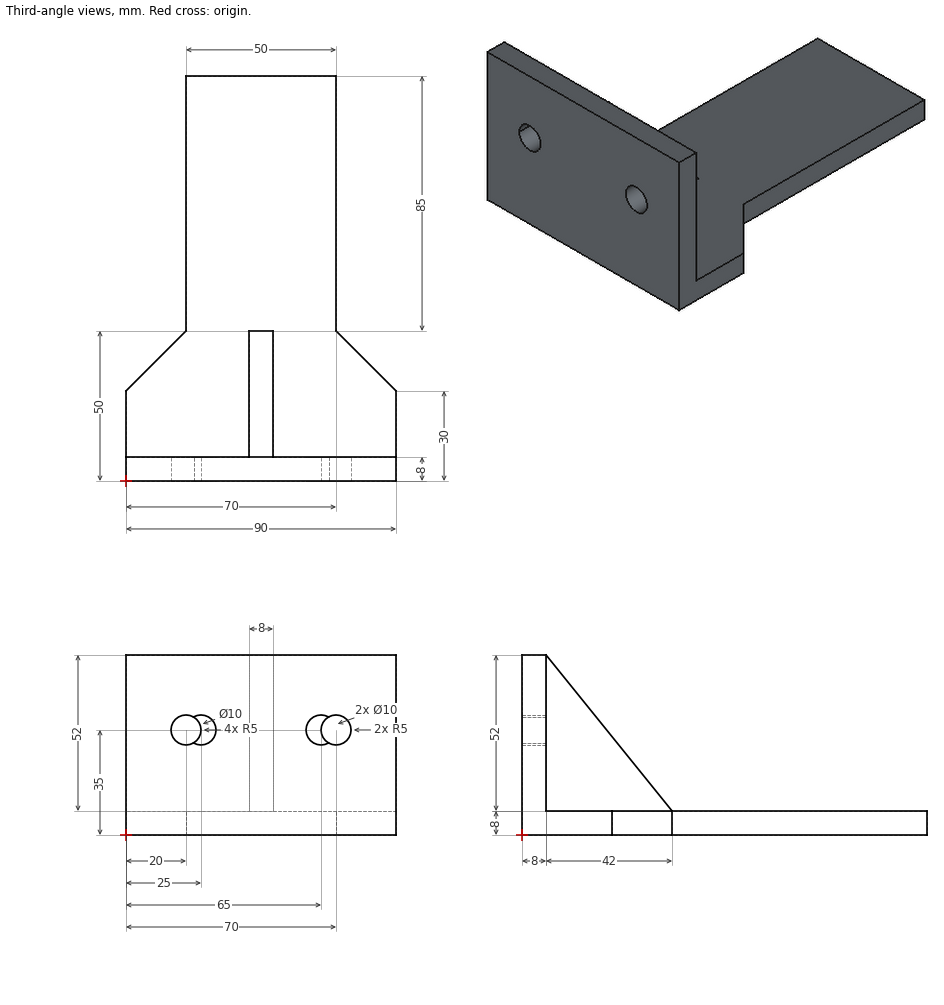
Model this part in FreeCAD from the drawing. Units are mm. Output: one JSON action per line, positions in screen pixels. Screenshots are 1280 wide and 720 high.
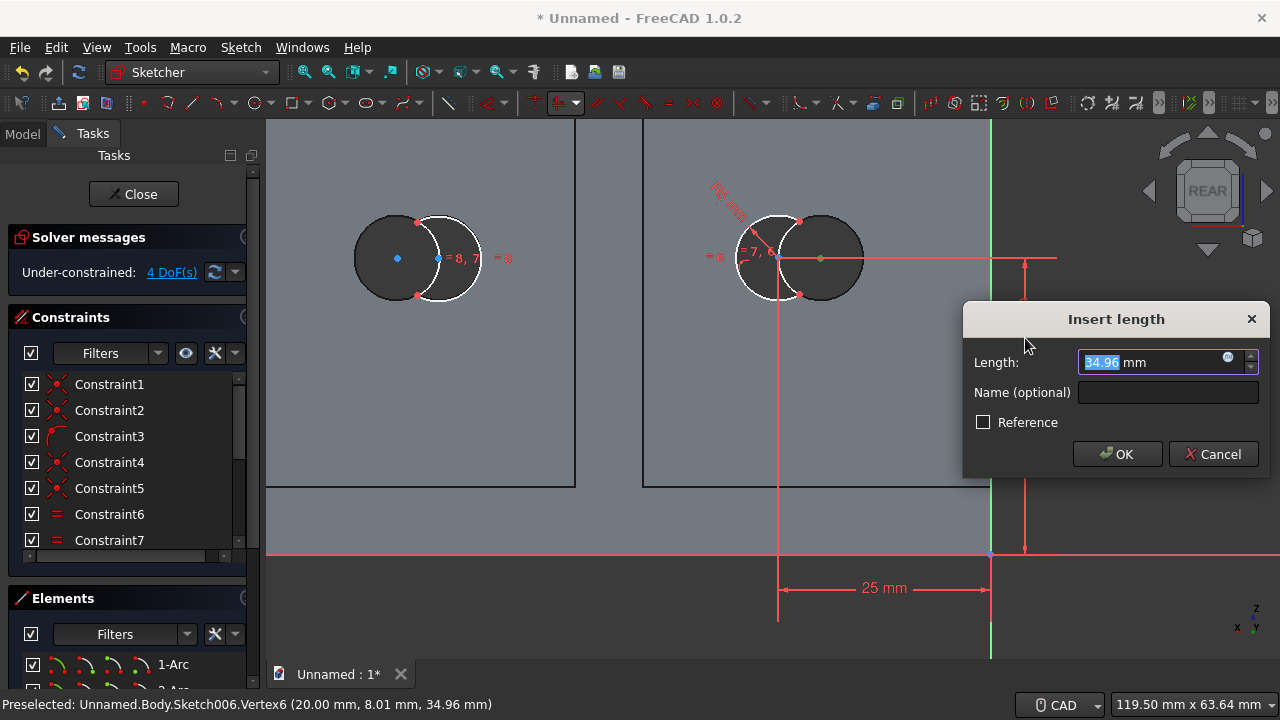
{"action": "type", "text": "35"}
{"action": "key", "text": "Return"}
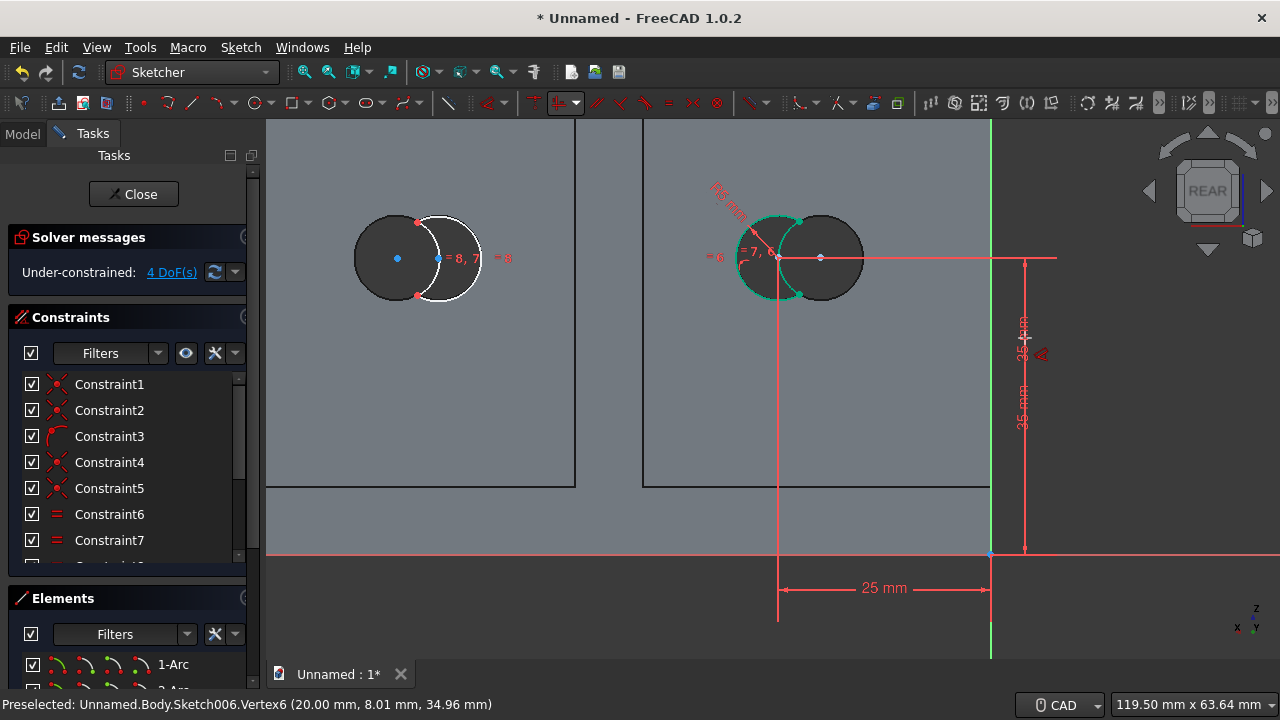
{"action": "left_click", "coordinate": [397, 259]}
{"action": "left_click", "coordinate": [694, 589]}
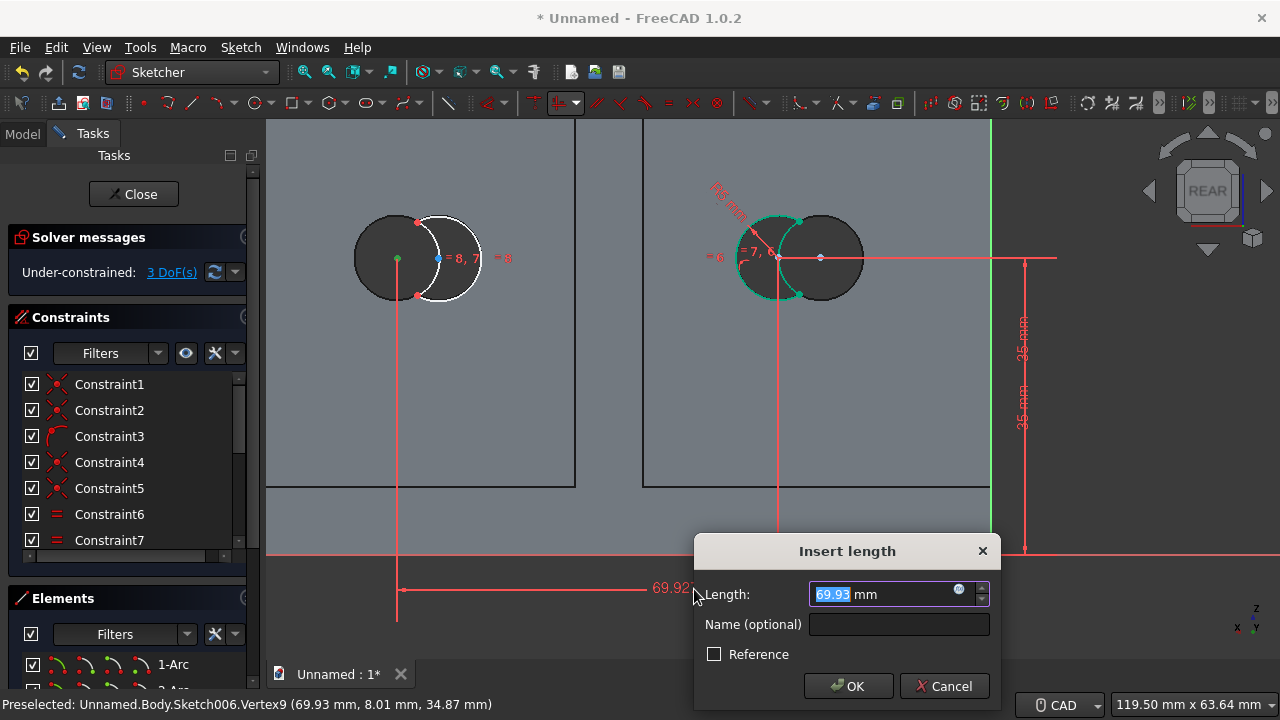
{"action": "type", "text": "70"}
{"action": "key", "text": "Return"}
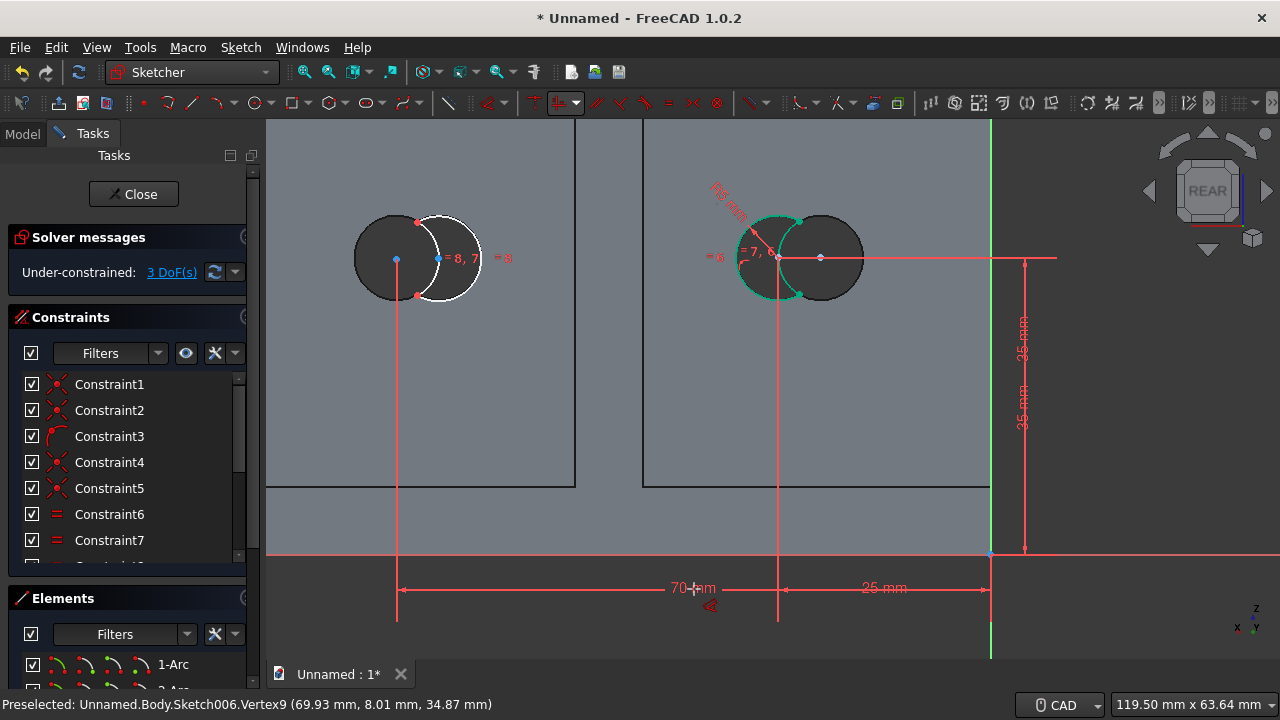
{"action": "left_click", "coordinate": [397, 259]}
{"action": "left_click", "coordinate": [363, 407]}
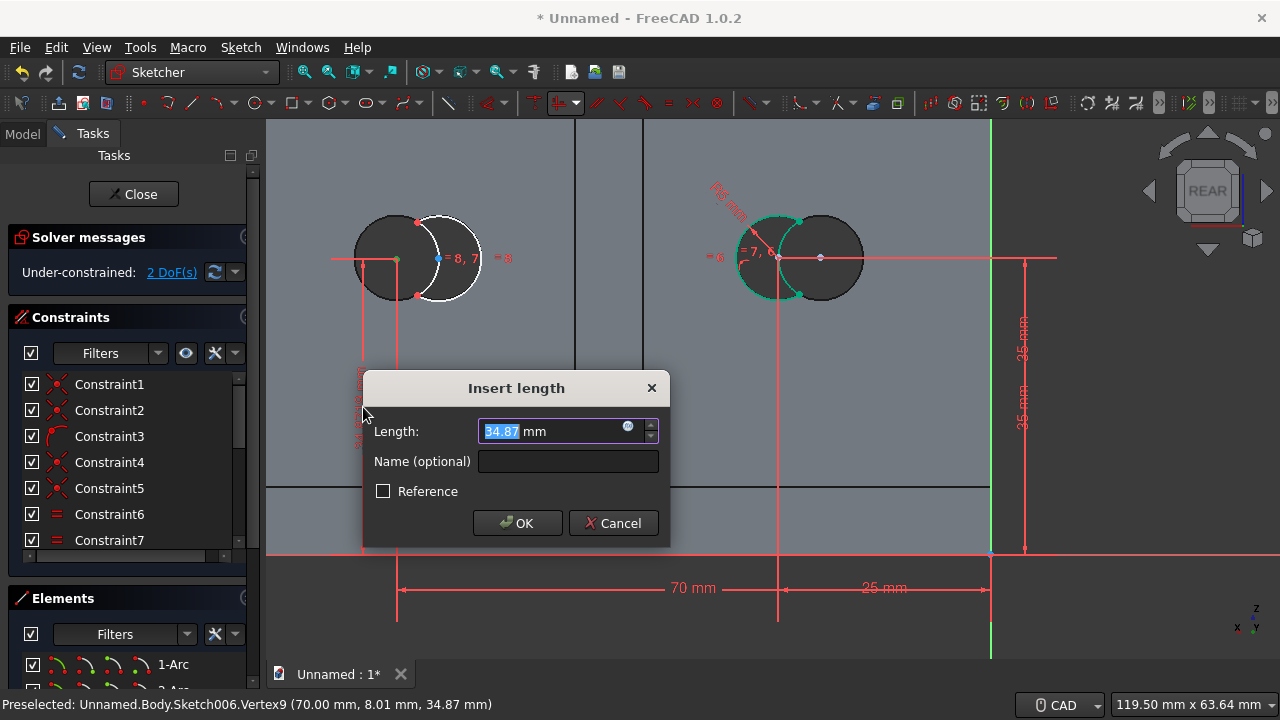
{"action": "type", "text": "35"}
{"action": "key", "text": "Return"}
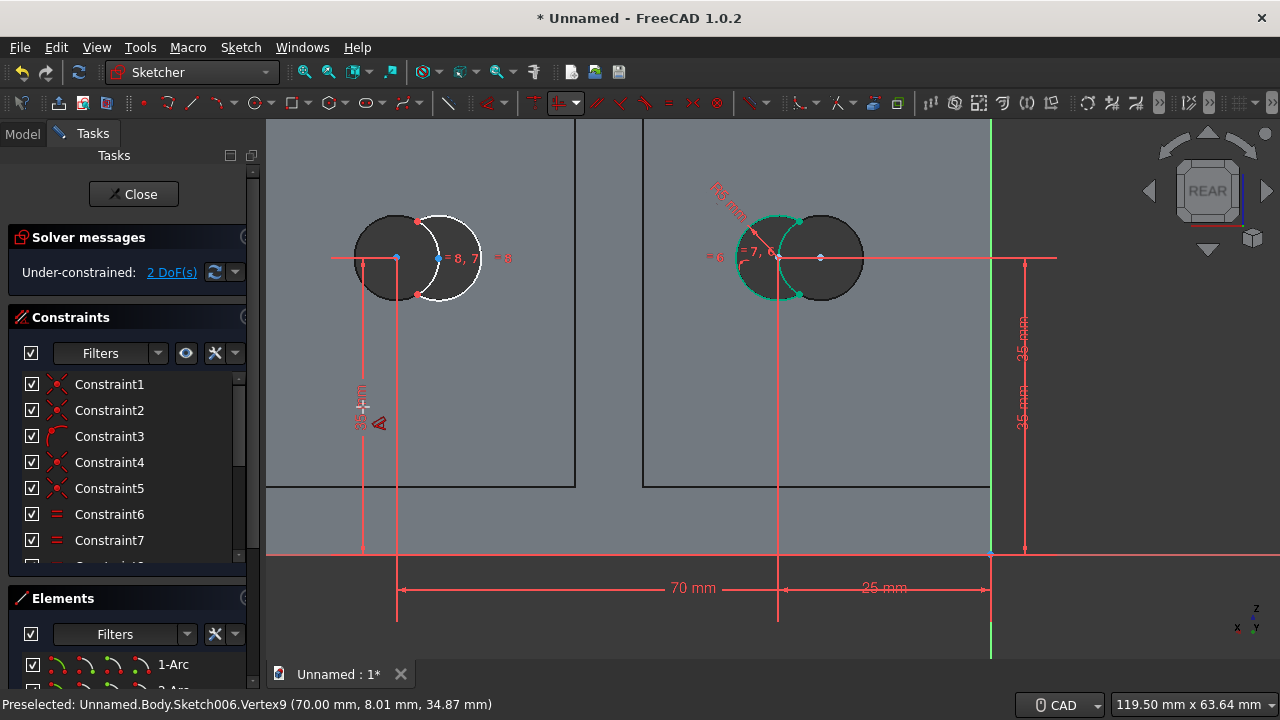
{"action": "left_click", "coordinate": [439, 258]}
{"action": "left_click", "coordinate": [588, 589]}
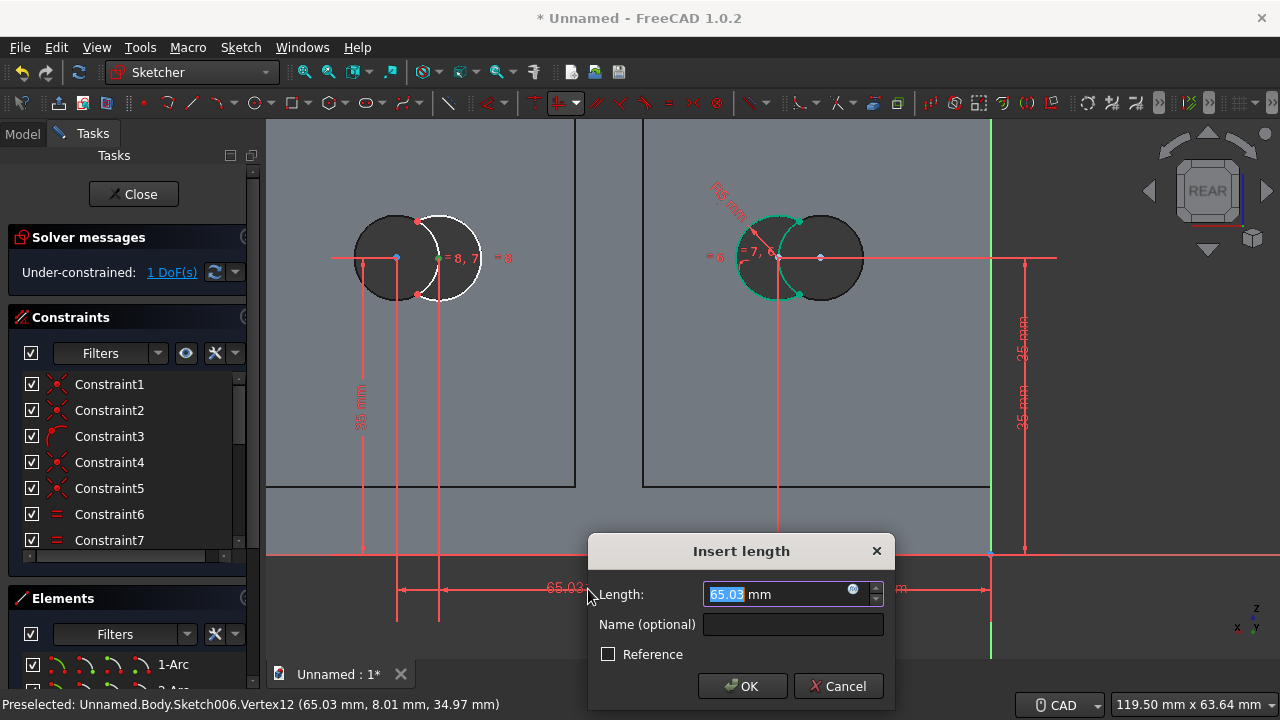
{"action": "type", "text": "65"}
{"action": "key", "text": "Return"}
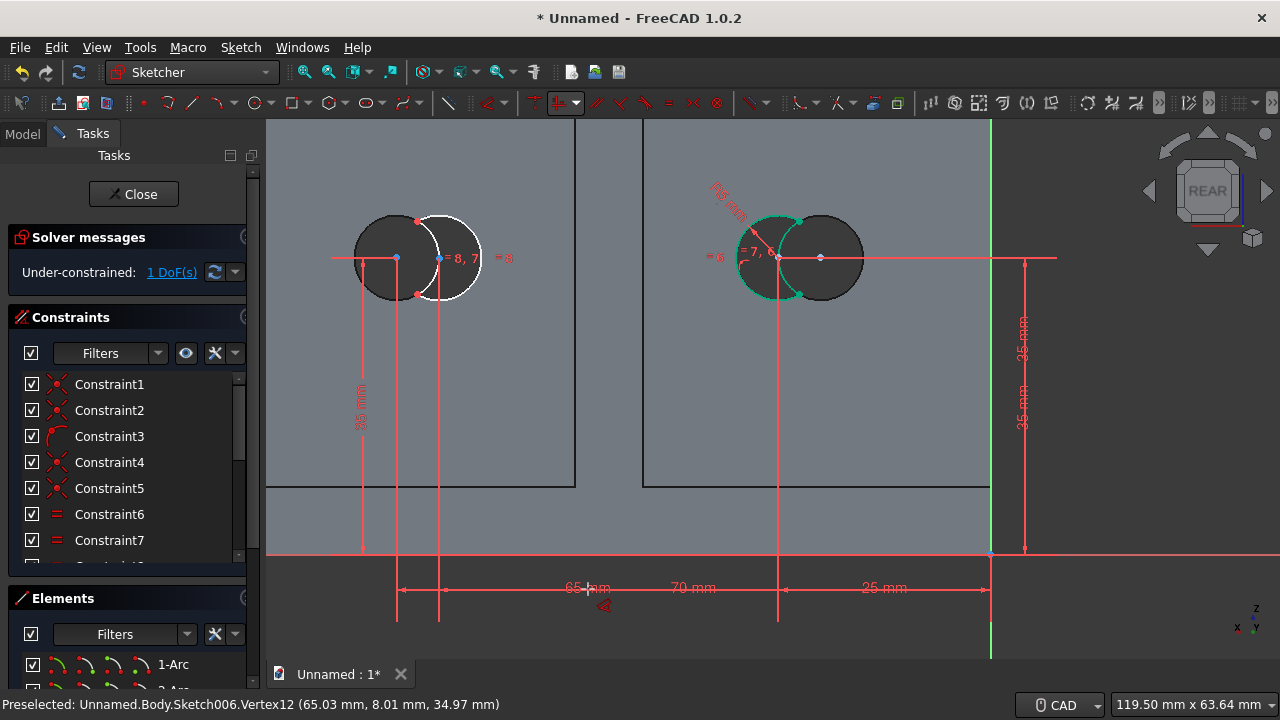
{"action": "left_click", "coordinate": [439, 258]}
{"action": "left_click", "coordinate": [1025, 475]}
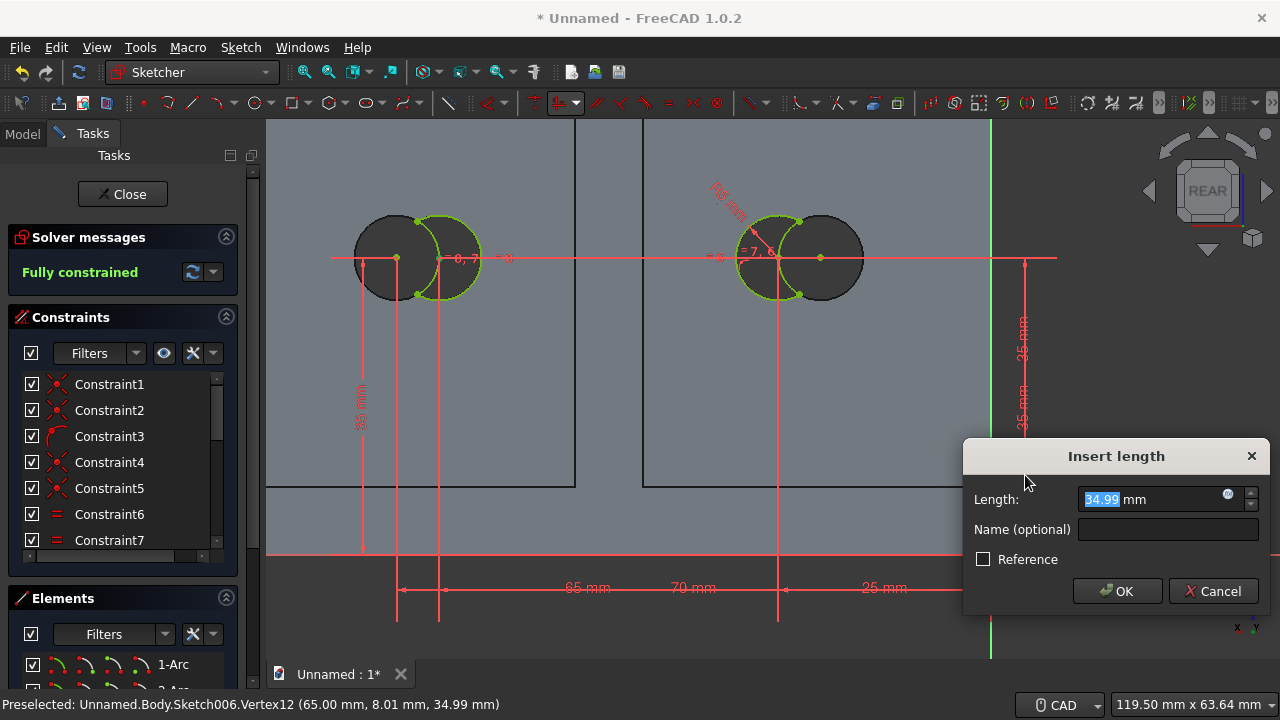
{"action": "type", "text": "35"}
{"action": "key", "text": "Return"}
{"action": "key", "text": "Escape"}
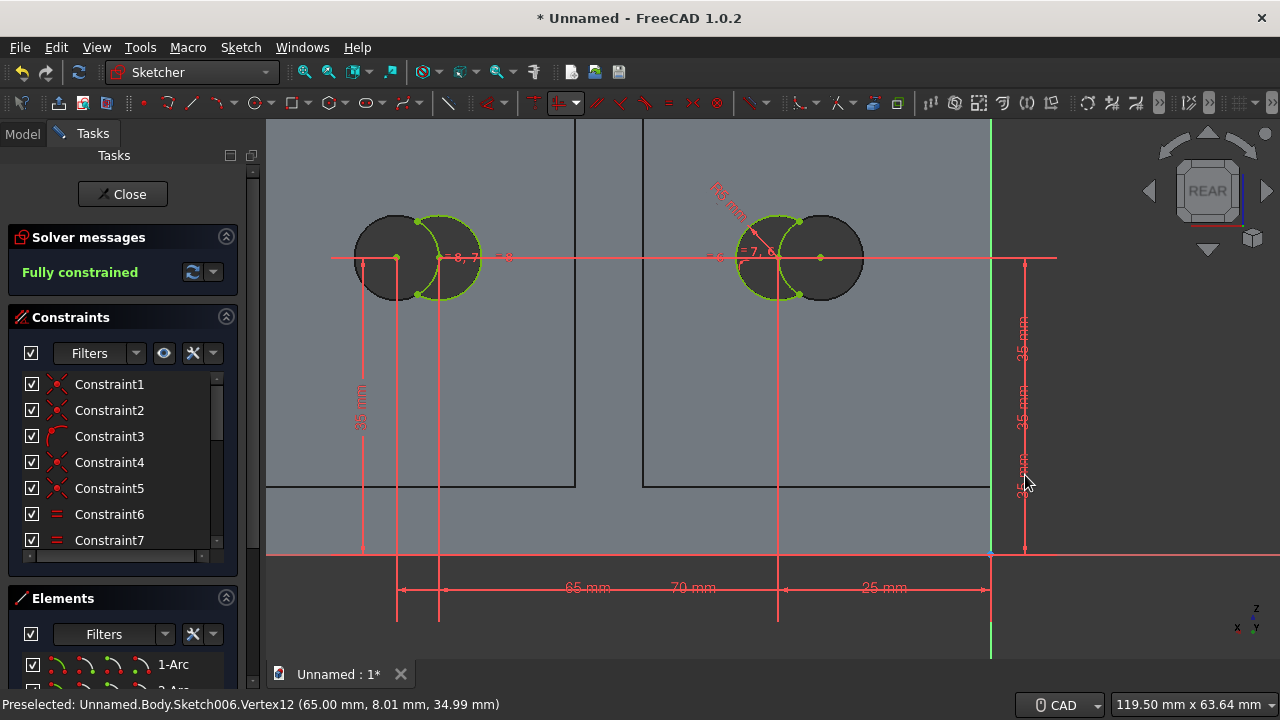
{"action": "left_click", "coordinate": [123, 194]}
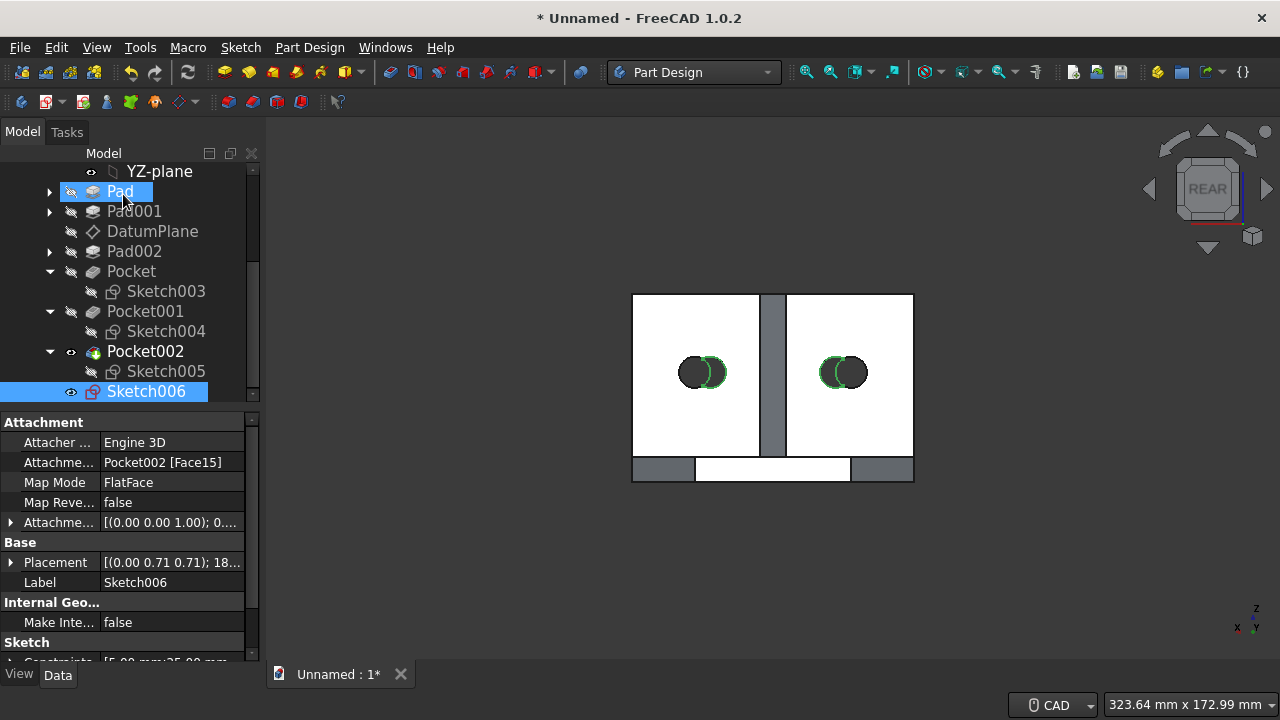
{"action": "left_click", "coordinate": [226, 72]}